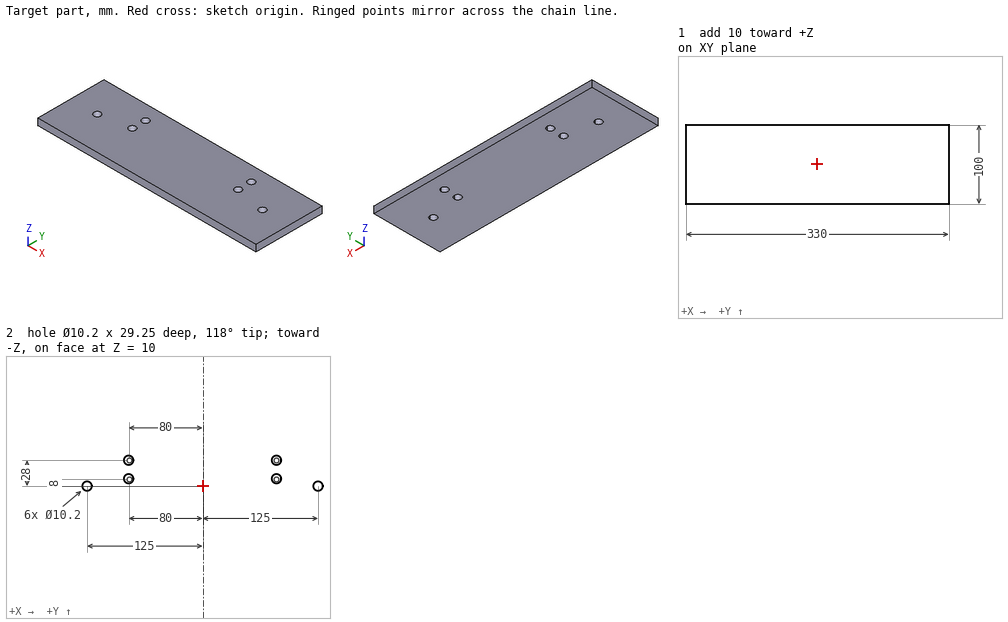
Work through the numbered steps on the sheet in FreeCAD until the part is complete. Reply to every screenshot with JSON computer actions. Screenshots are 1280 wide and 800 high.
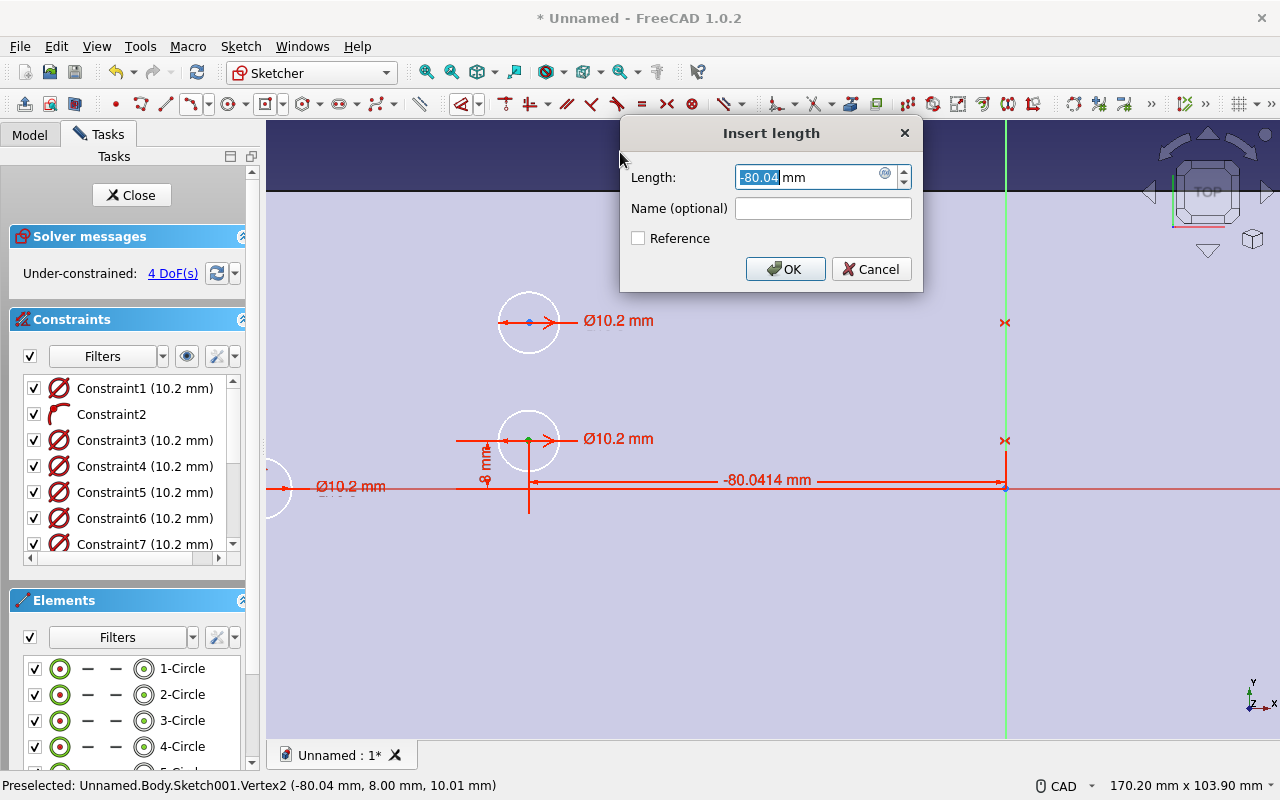
{"action": "type", "text": "-80"}
{"action": "key", "text": "Return"}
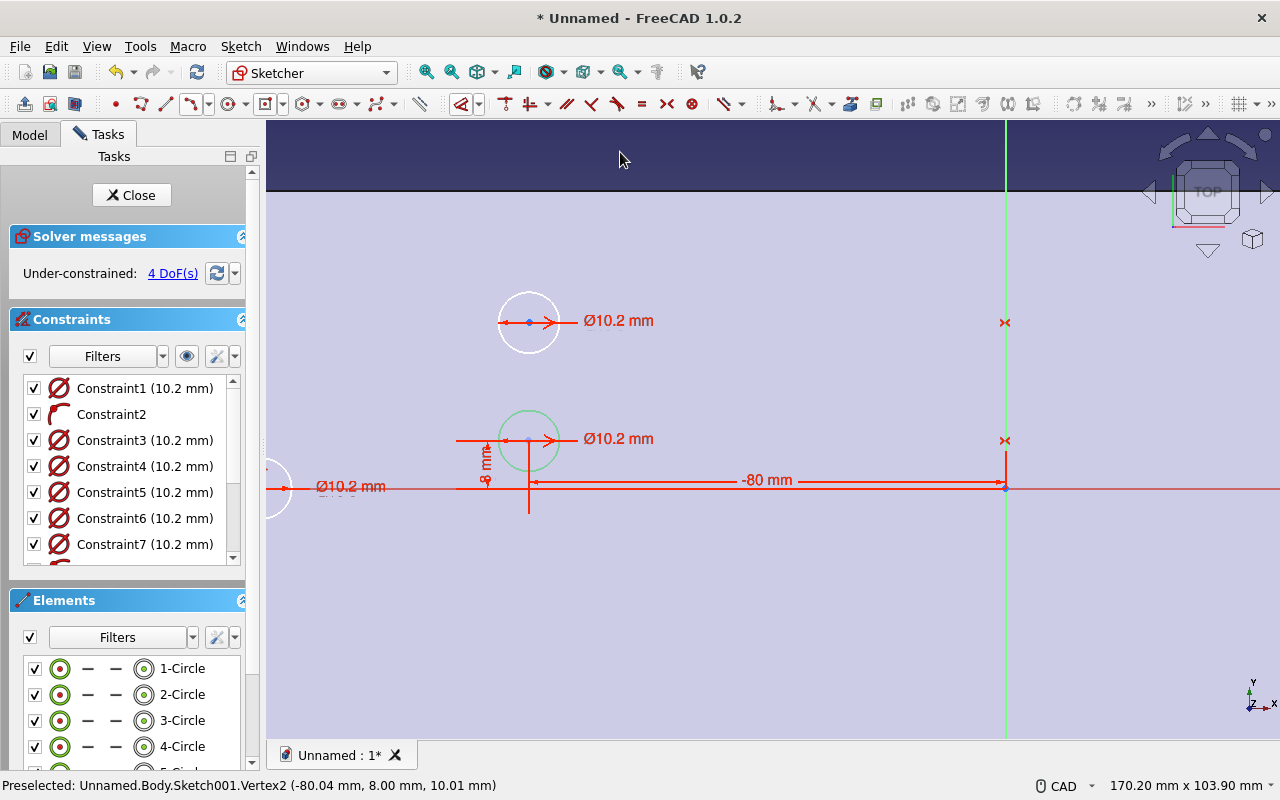
{"action": "left_click", "coordinate": [529, 323]}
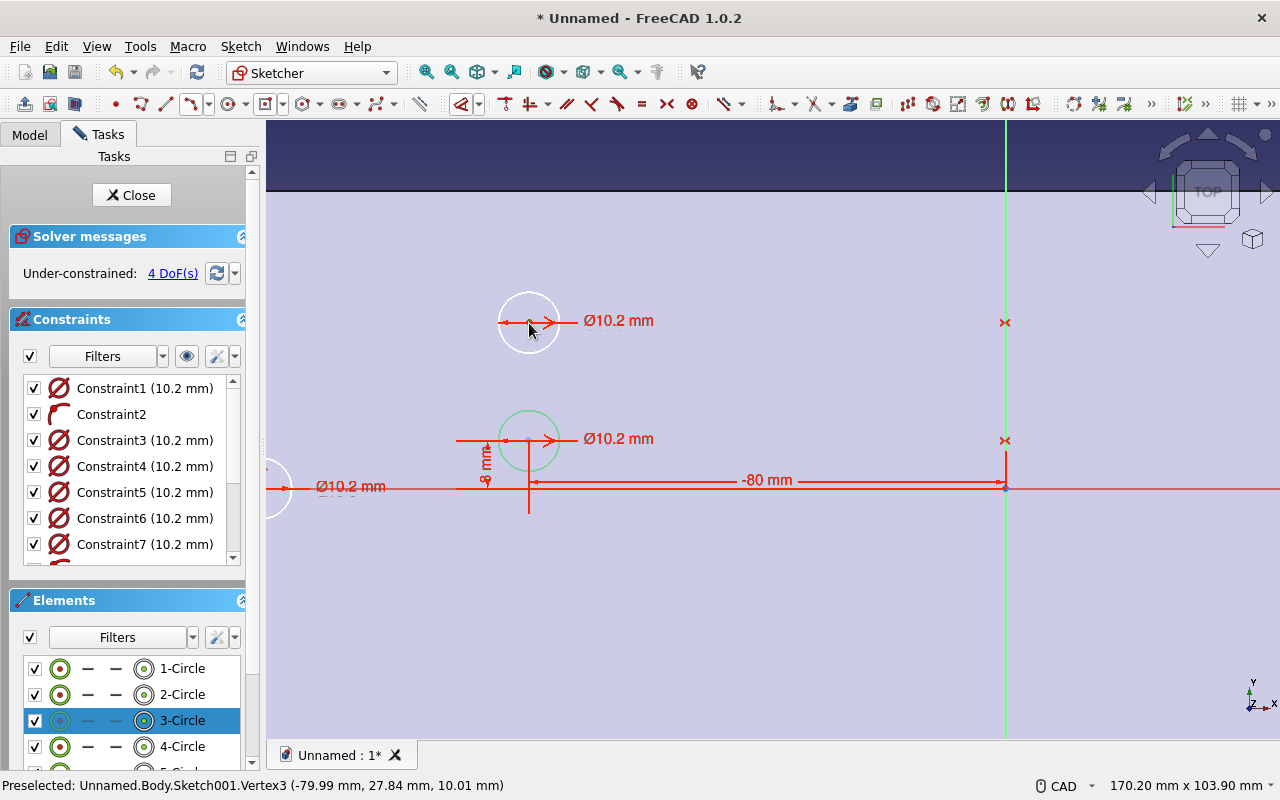
{"action": "left_click", "coordinate": [478, 104]}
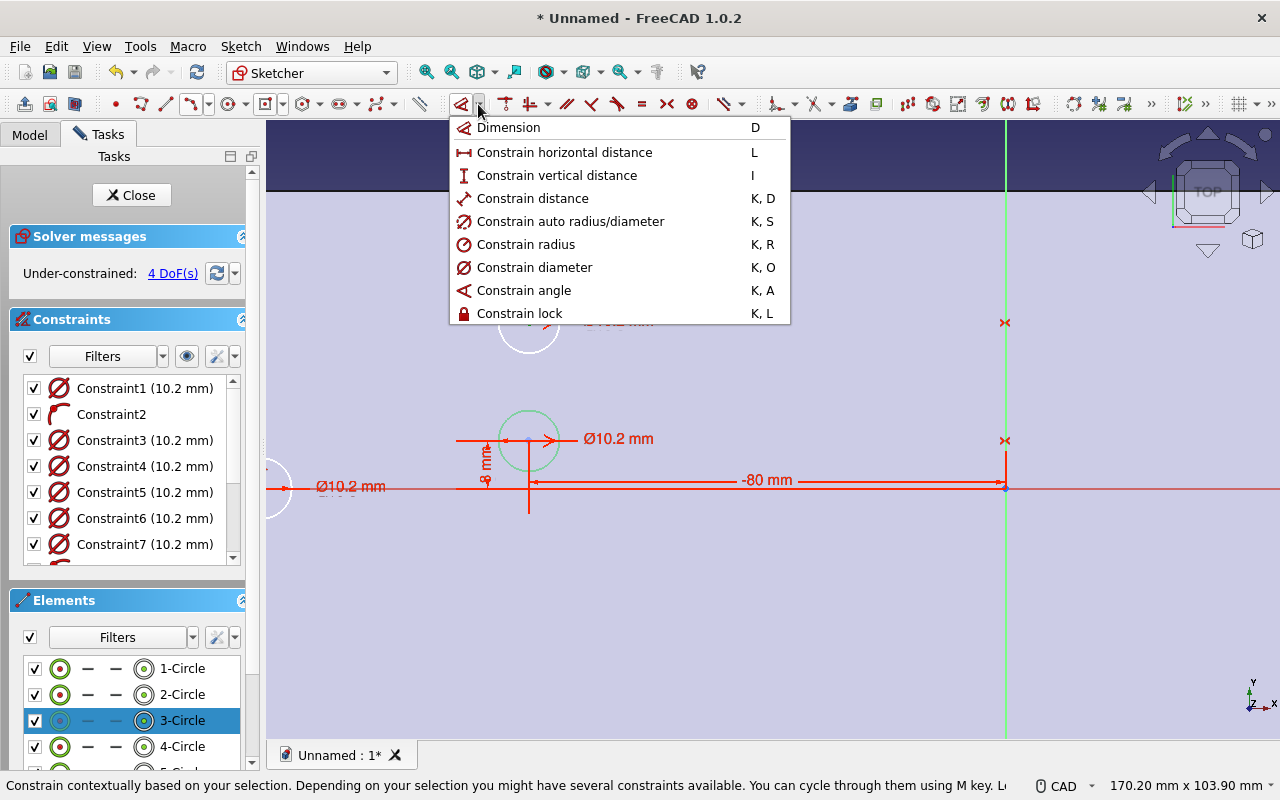
{"action": "left_click", "coordinate": [620, 152]}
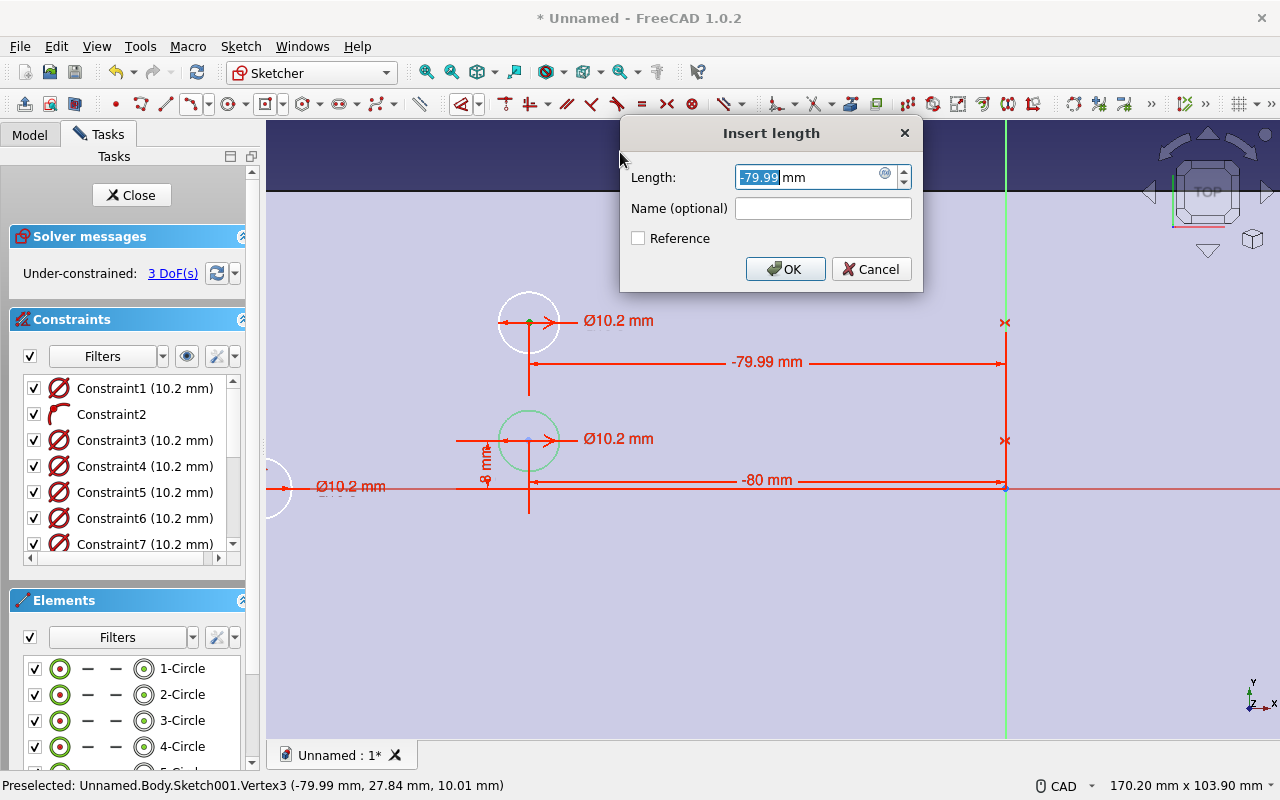
{"action": "type", "text": "-80"}
{"action": "key", "text": "Return"}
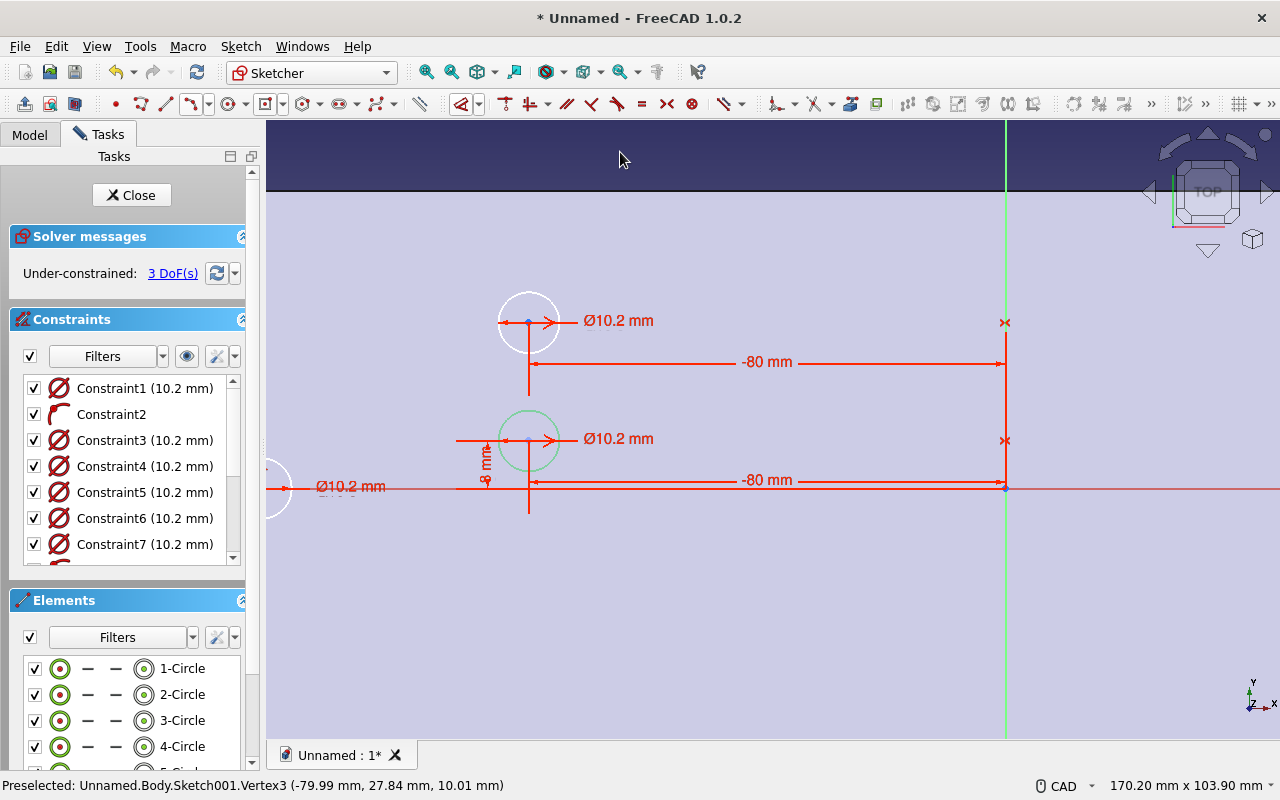
{"action": "left_click", "coordinate": [529, 323]}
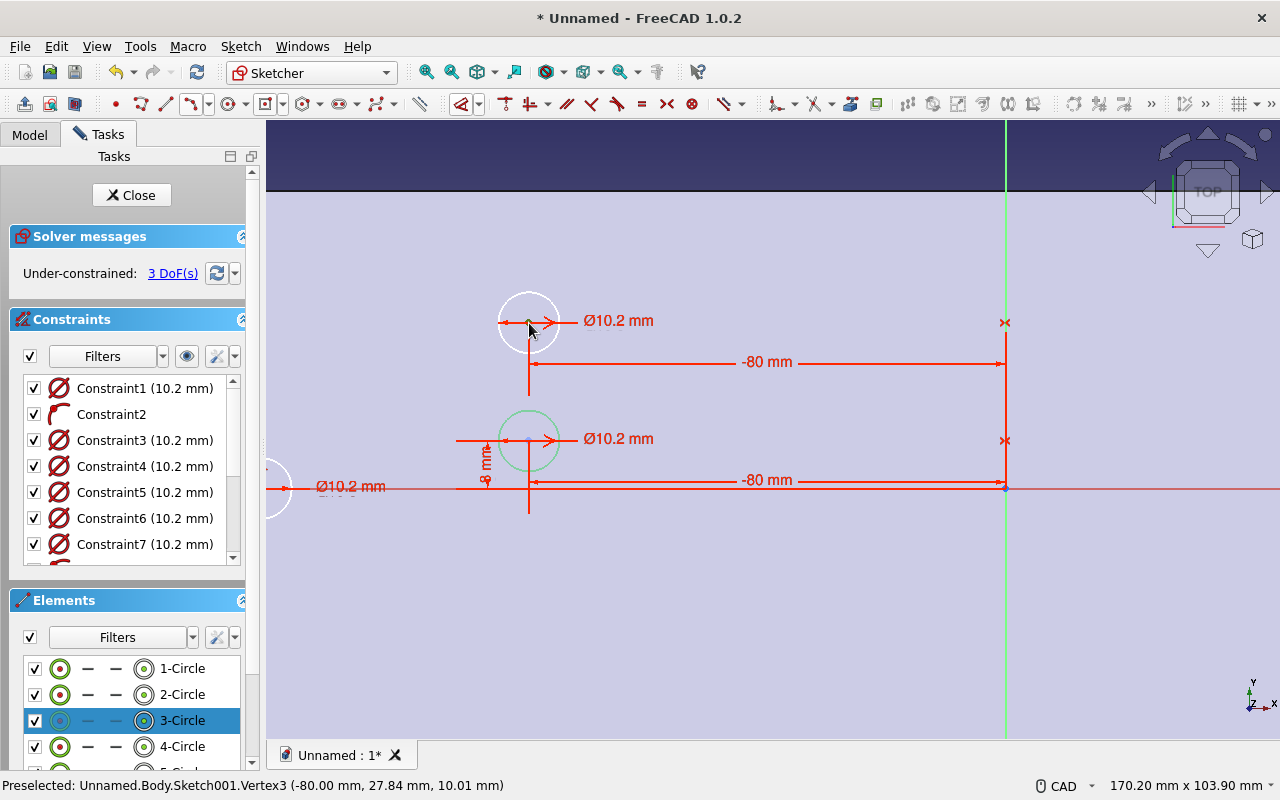
{"action": "left_click", "coordinate": [478, 104]}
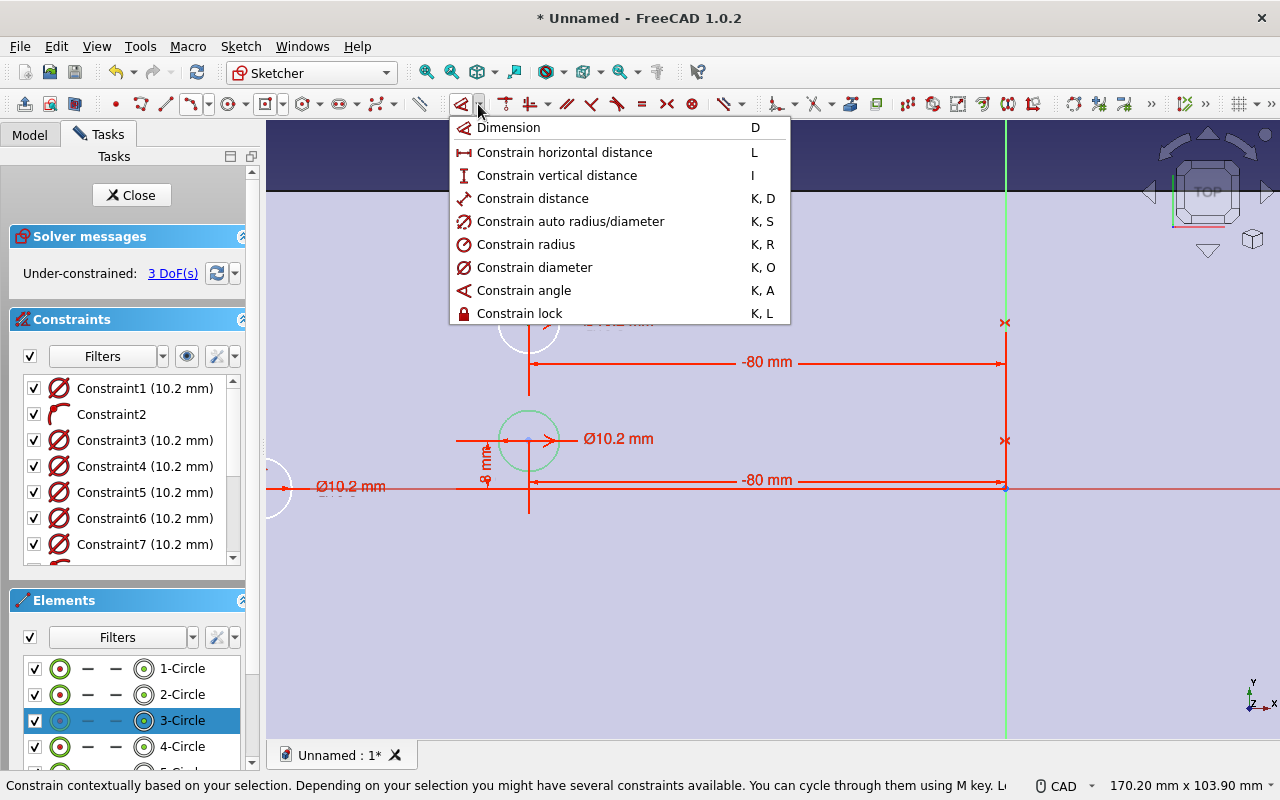
{"action": "left_click", "coordinate": [620, 176]}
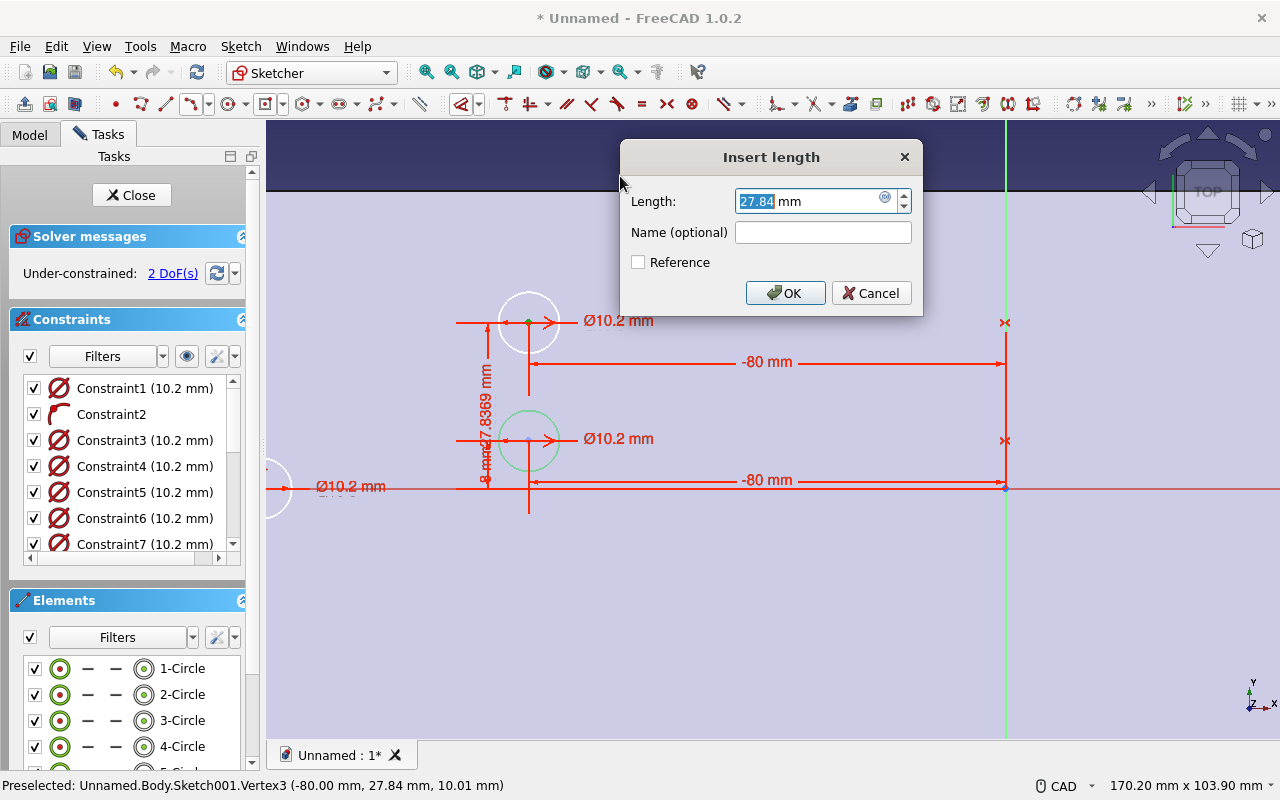
{"action": "type", "text": "28"}
{"action": "key", "text": "Return"}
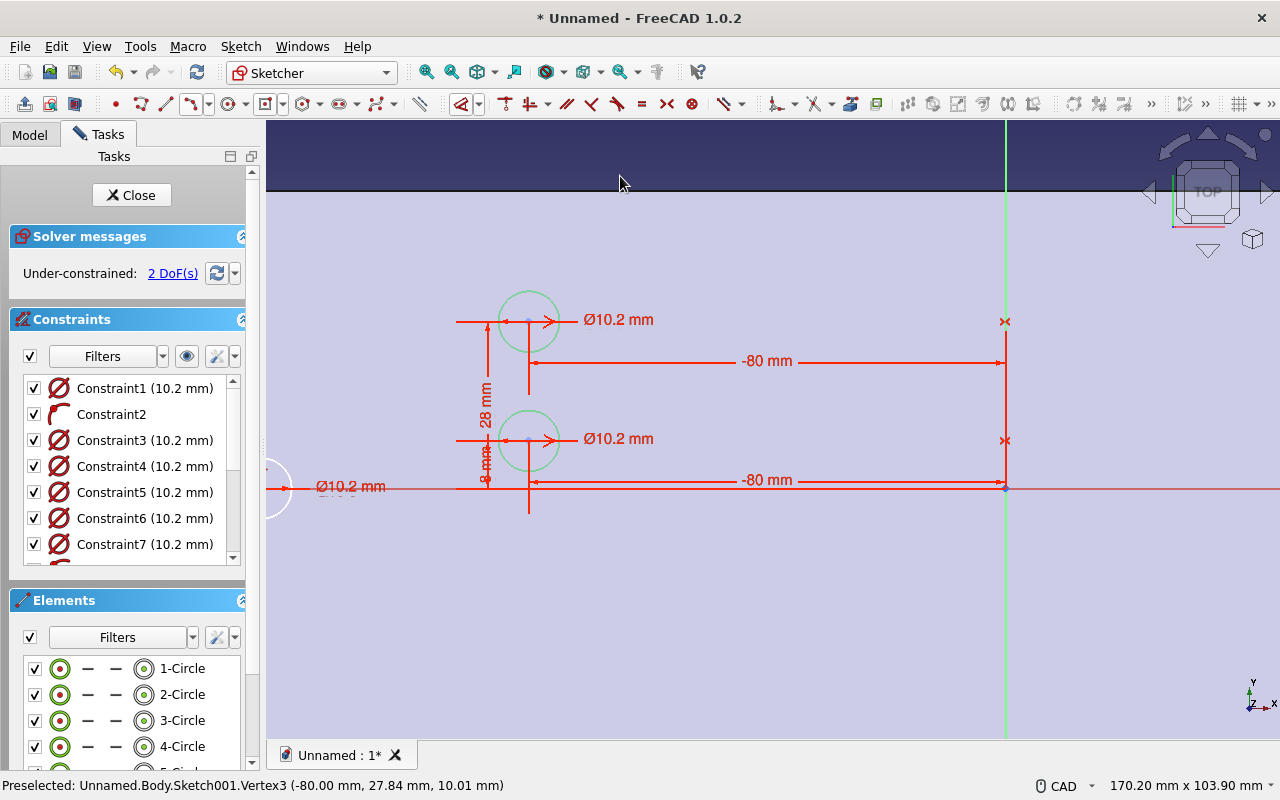
{"action": "scroll", "coordinate": [529, 444], "scroll_direction": "down", "scroll_amount": 5}